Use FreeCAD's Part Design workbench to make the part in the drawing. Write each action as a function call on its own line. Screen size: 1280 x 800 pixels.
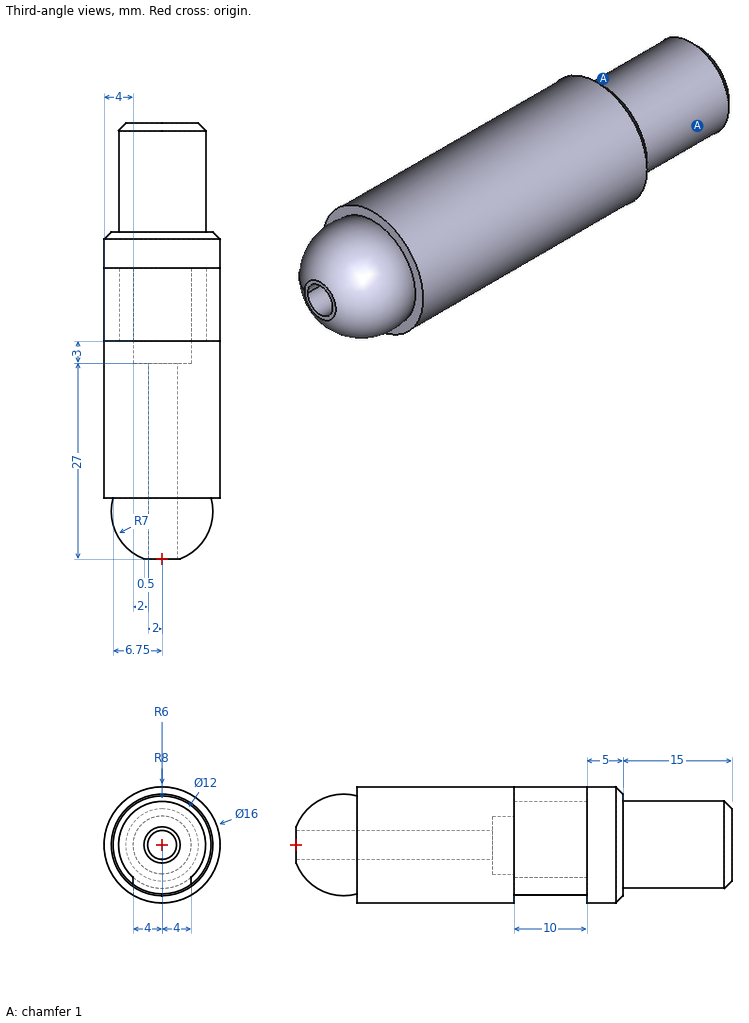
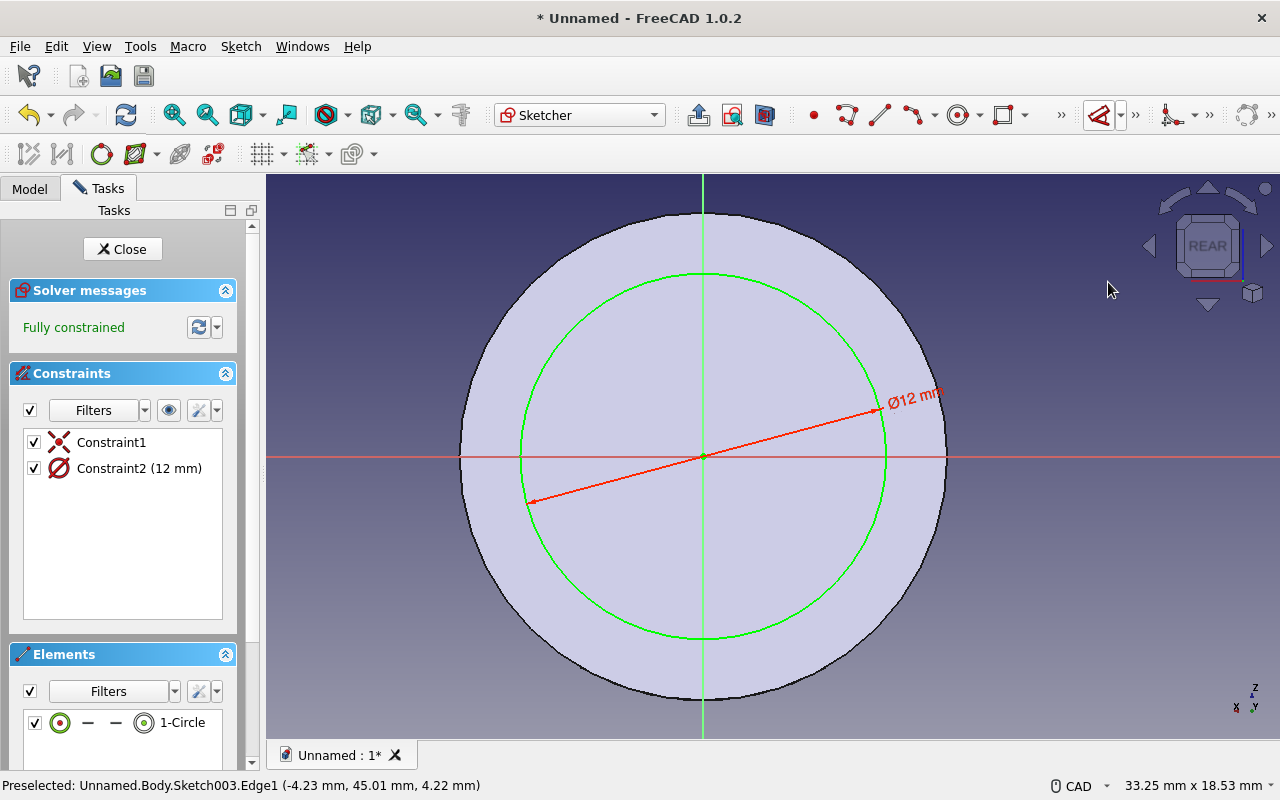
click(123, 249)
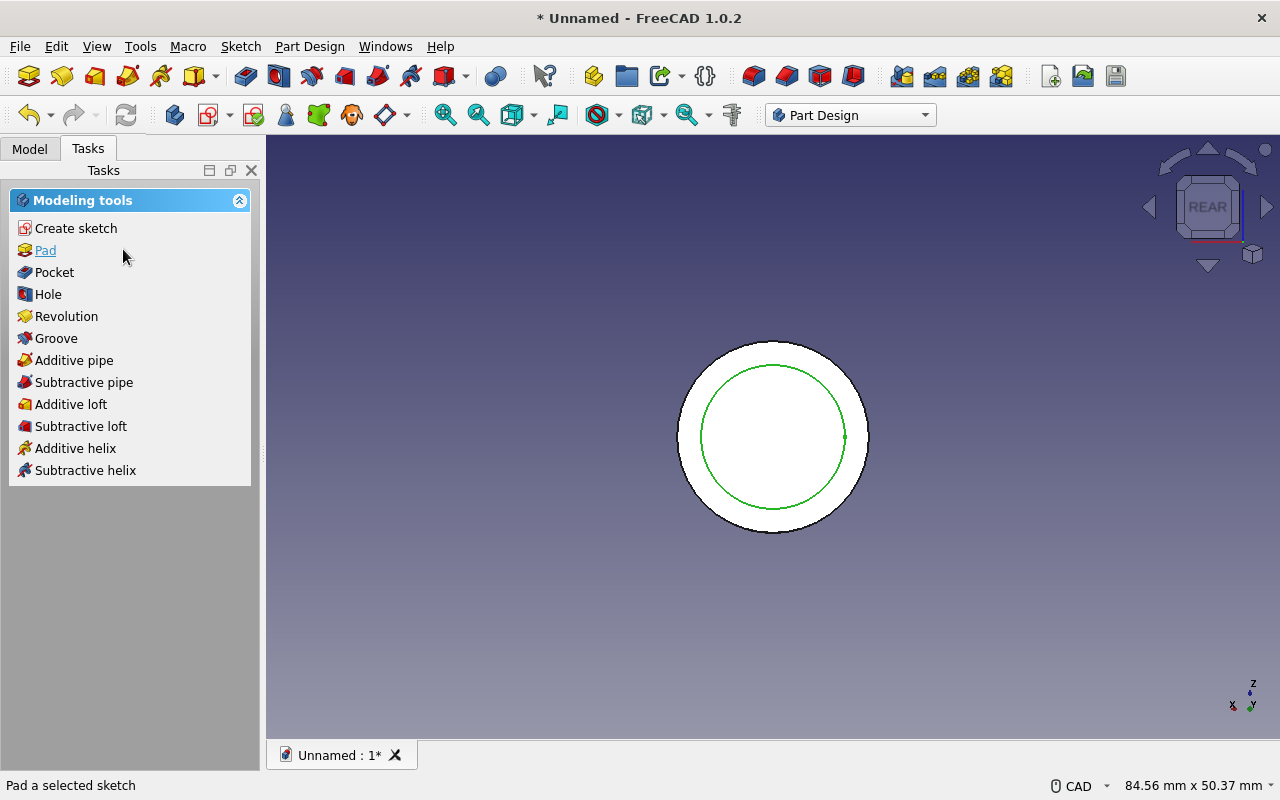
click(29, 76)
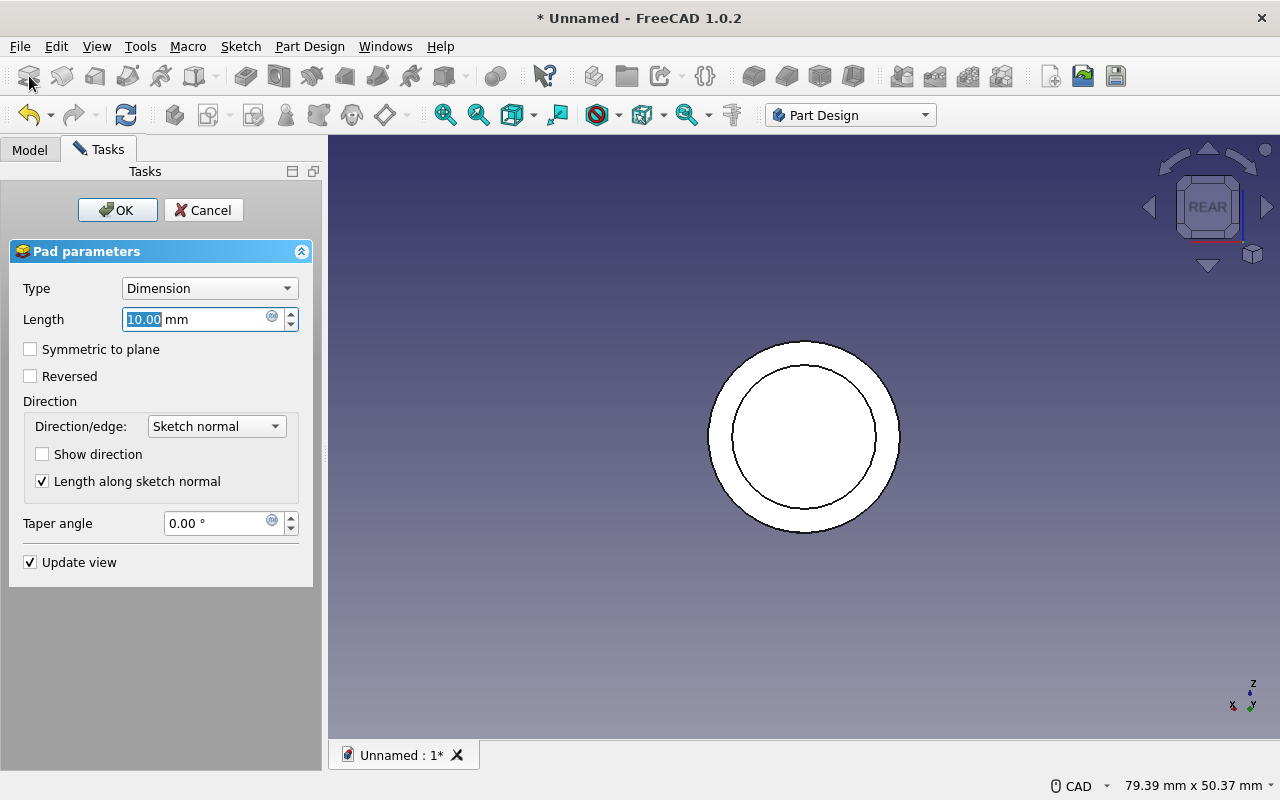
text(15)
key(Tab)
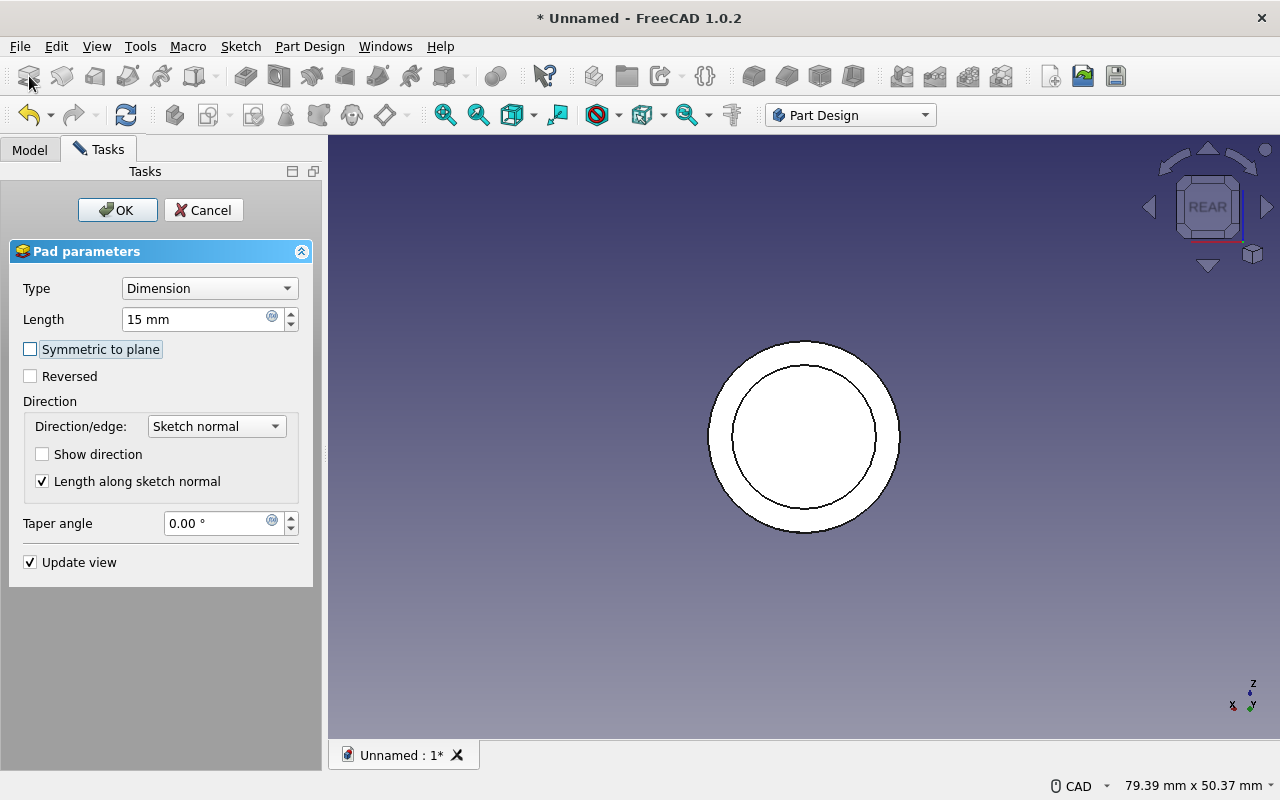
click(118, 210)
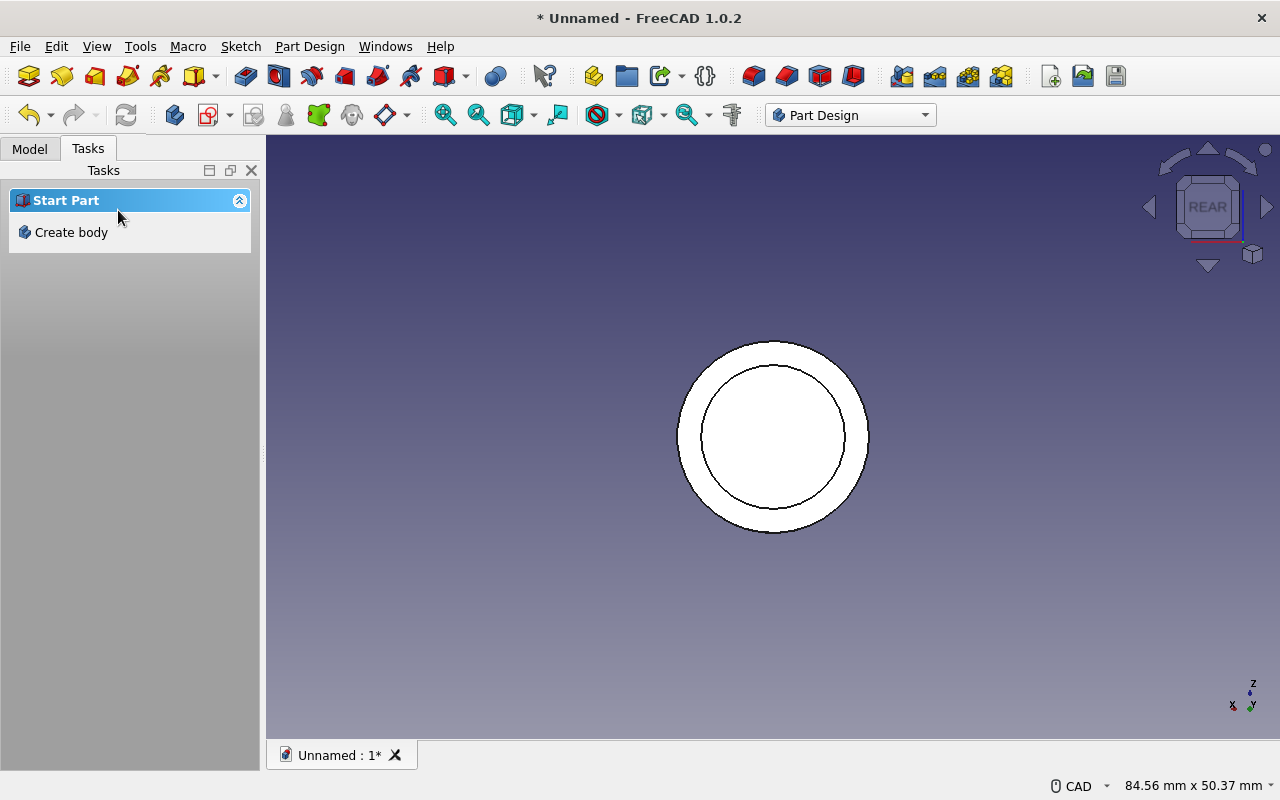
click(446, 116)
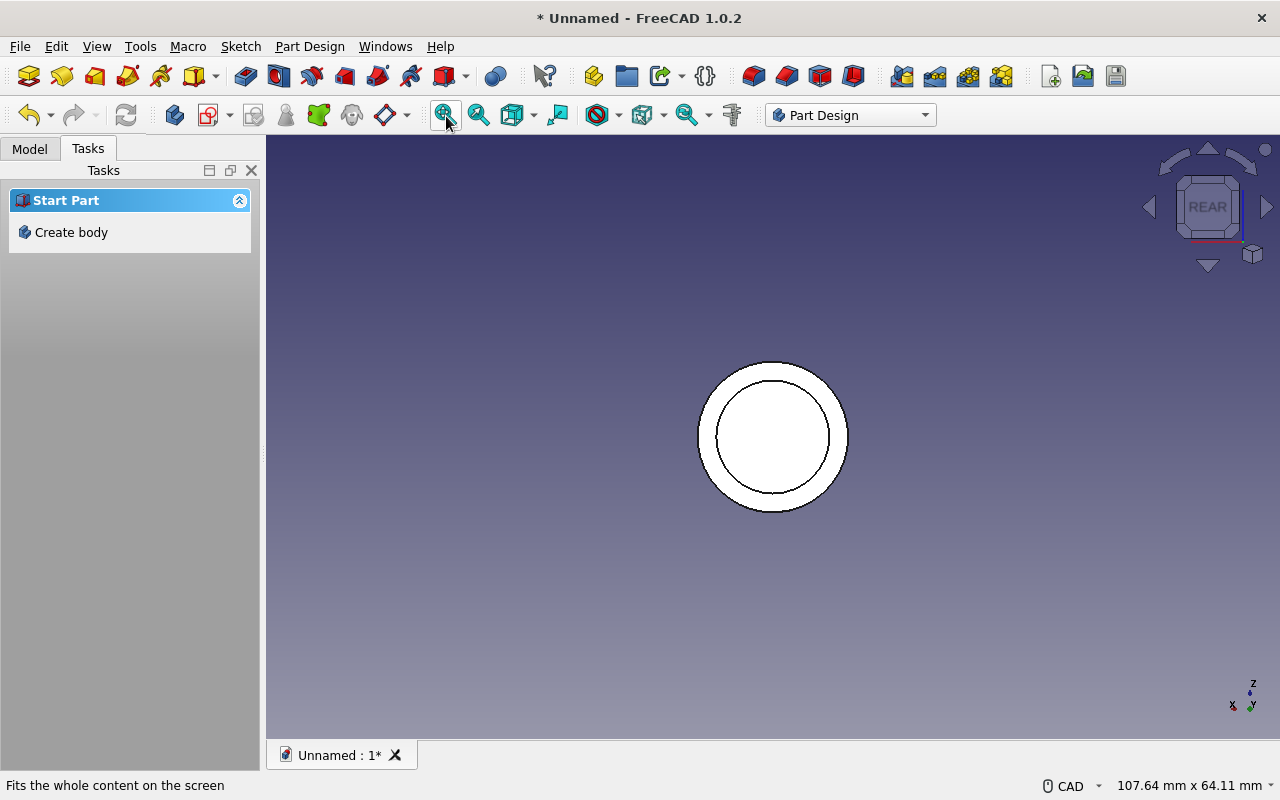
click(796, 364)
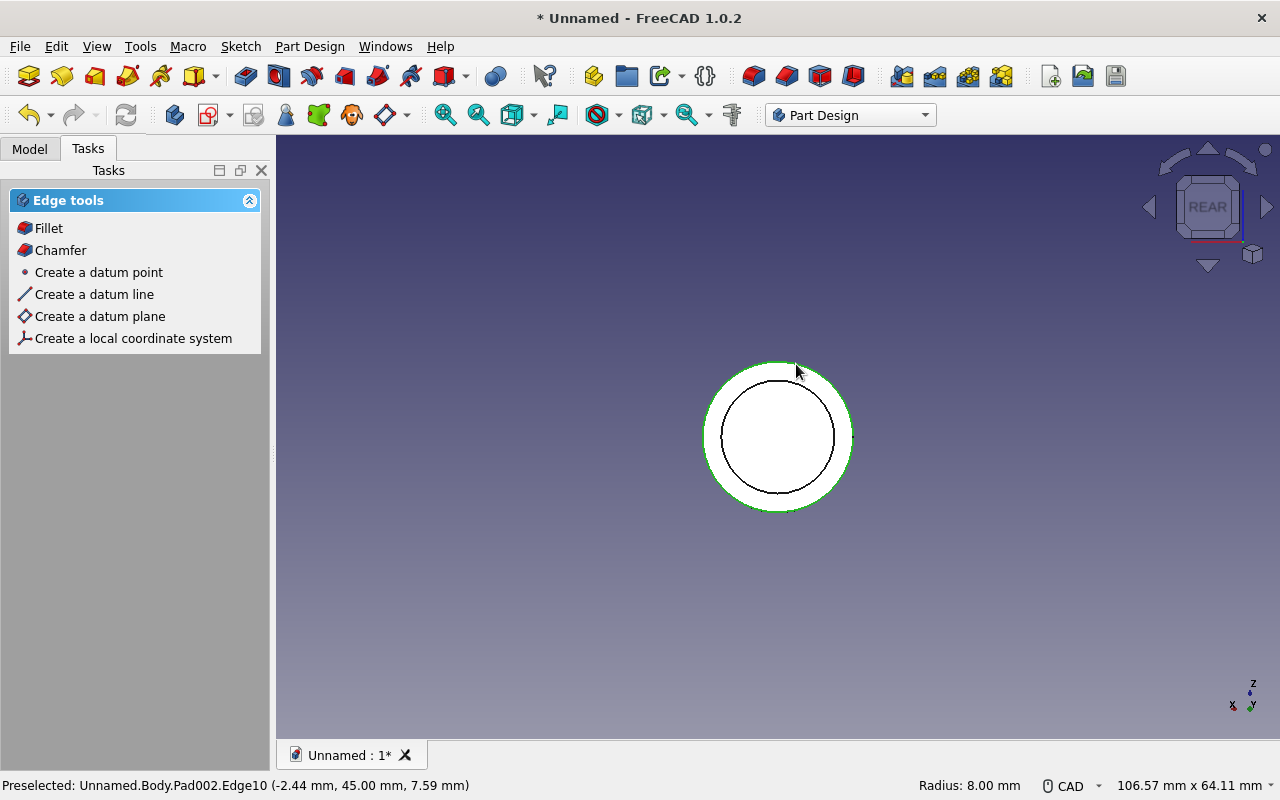
click(795, 382, ctrl)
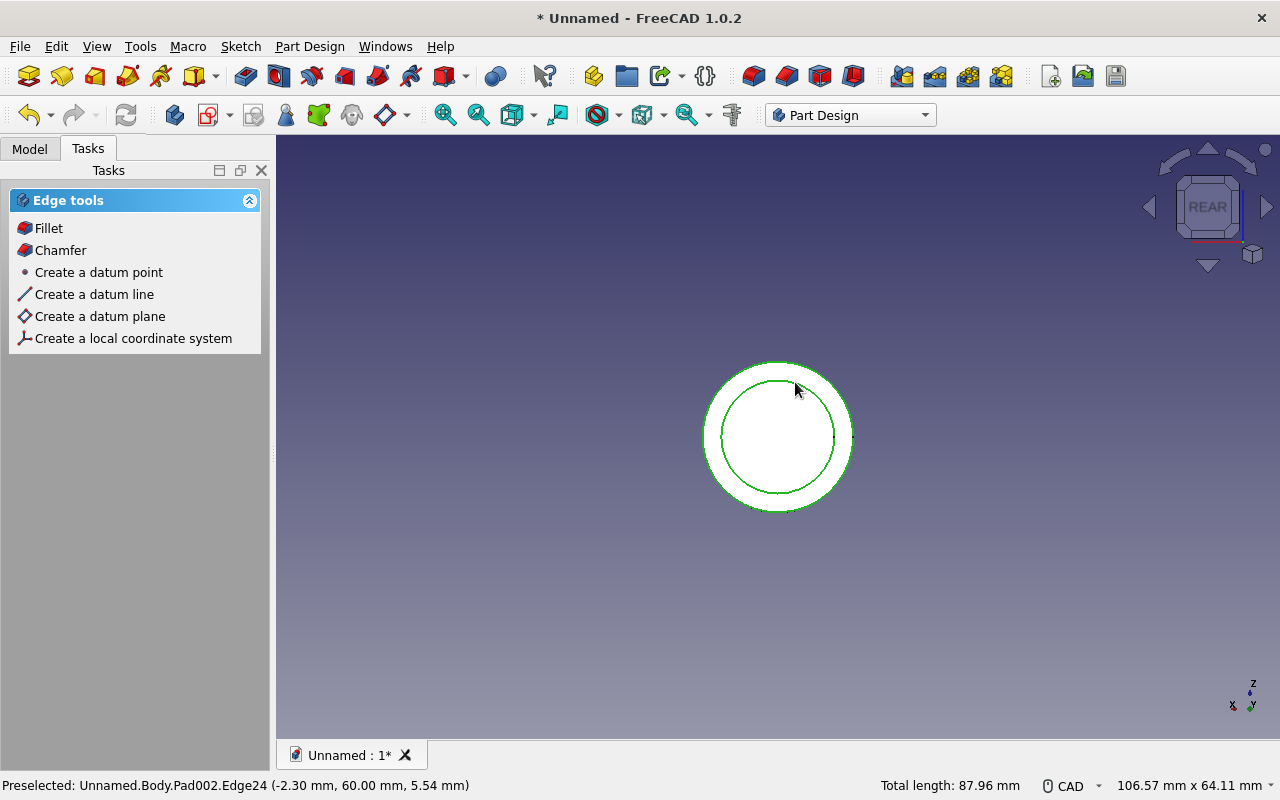
click(787, 76)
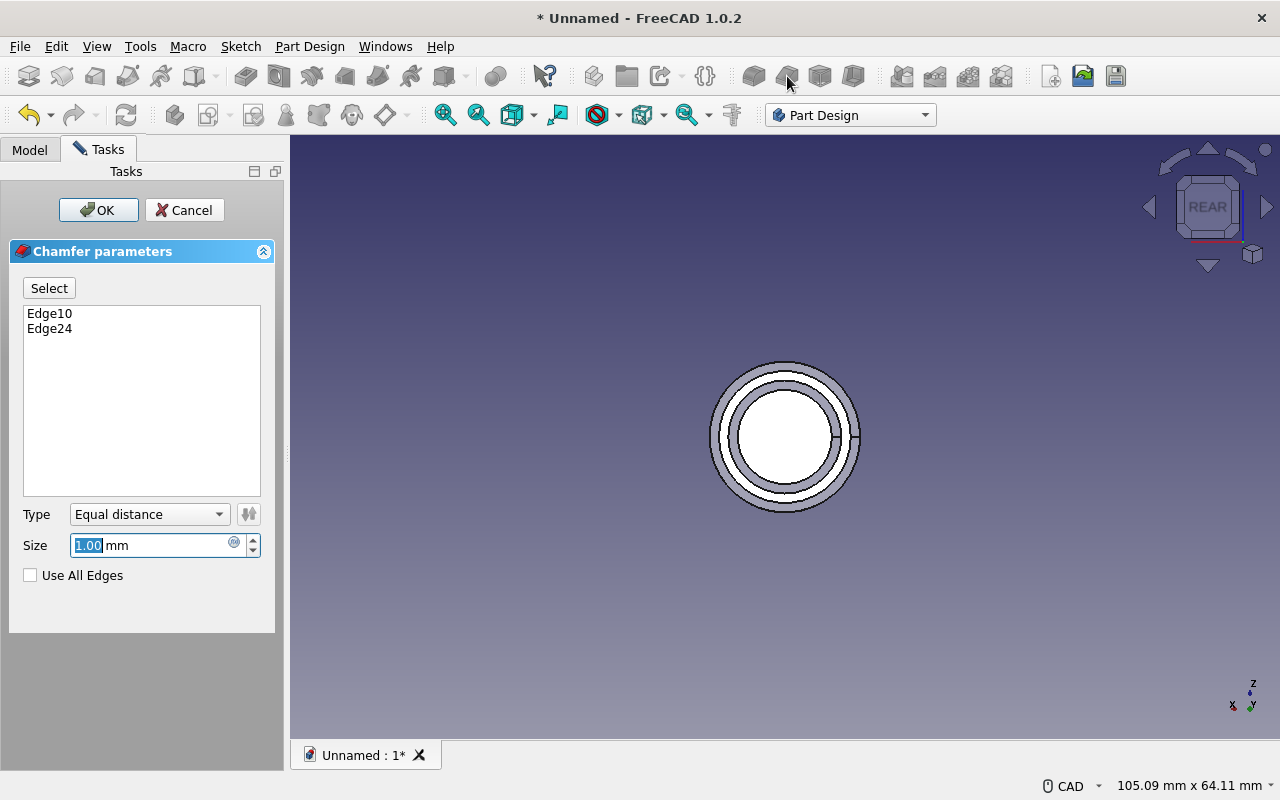
text(1)
key(Tab)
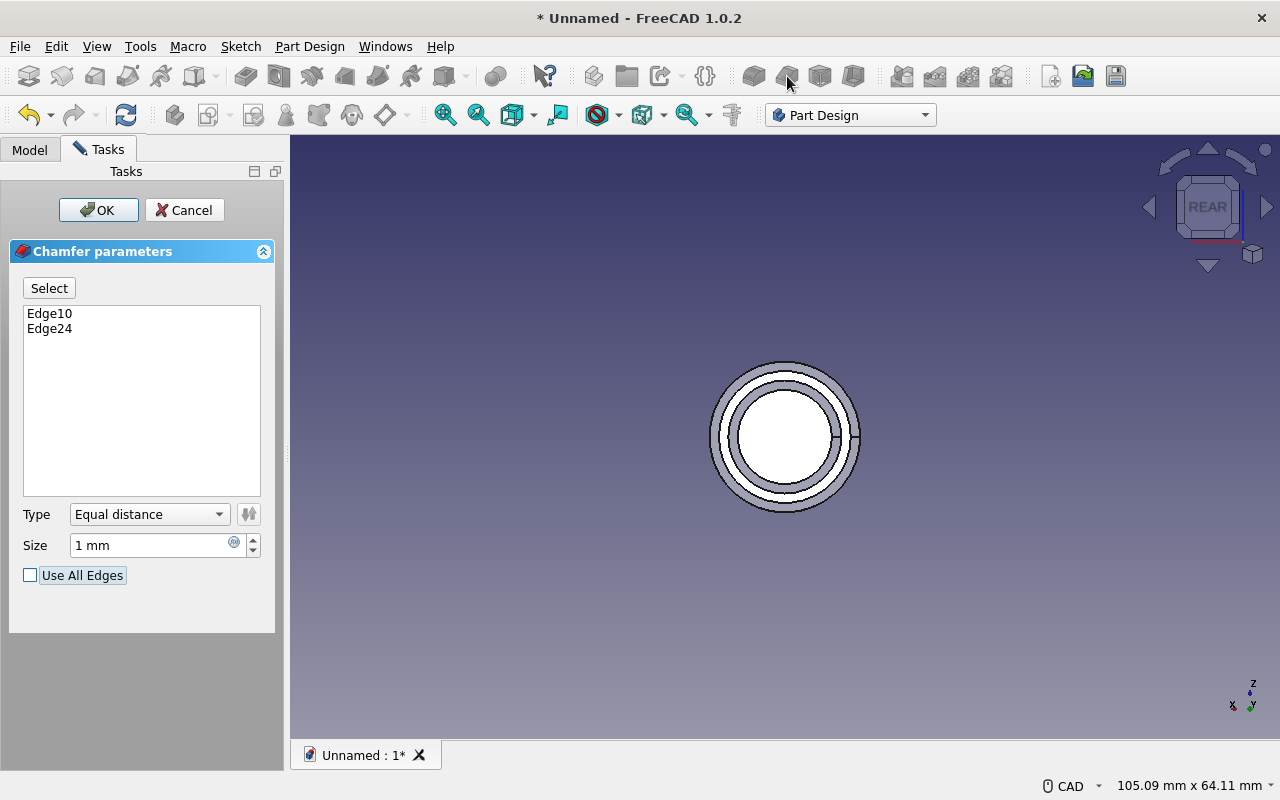
click(99, 210)